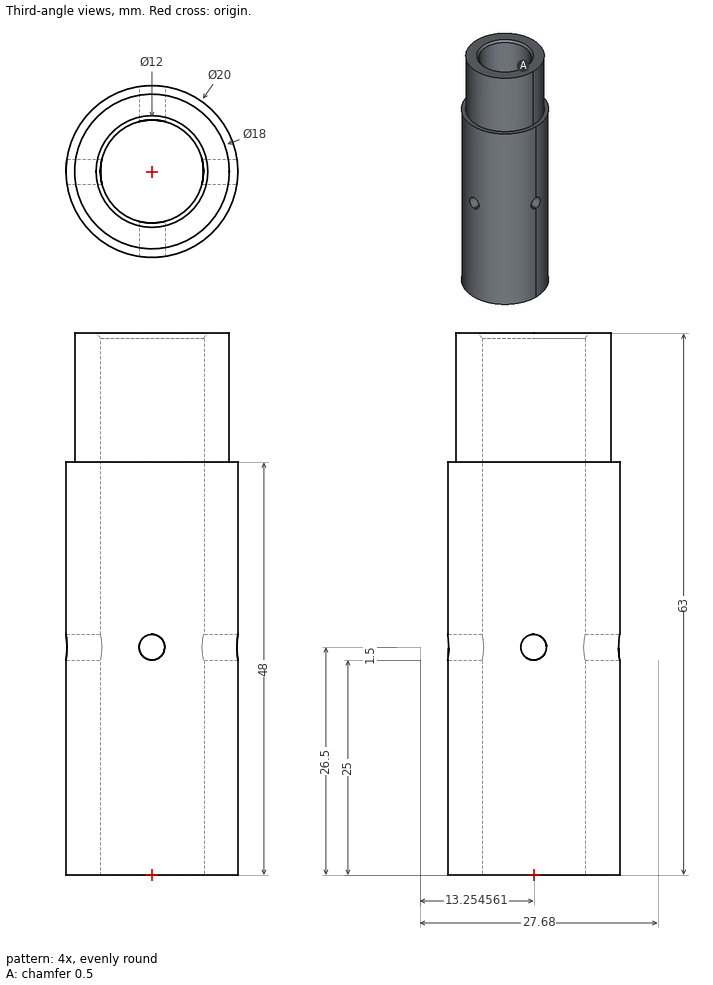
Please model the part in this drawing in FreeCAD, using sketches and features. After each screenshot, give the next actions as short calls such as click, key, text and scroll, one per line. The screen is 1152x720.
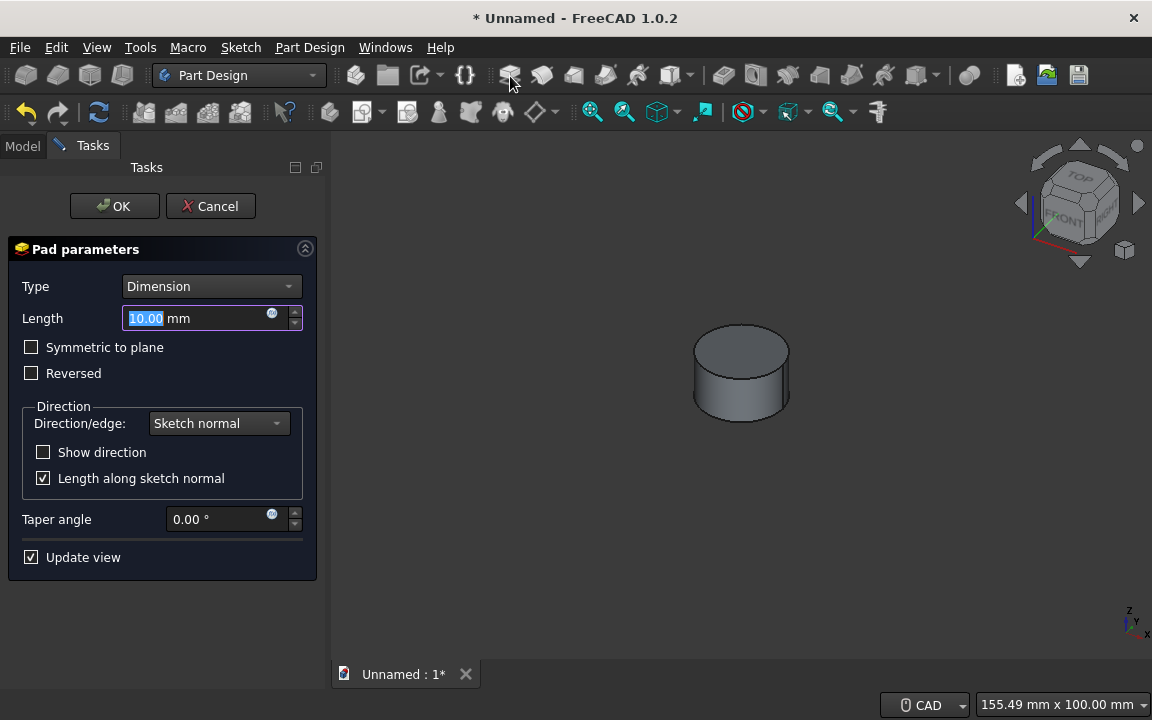
text(63)
key(Tab)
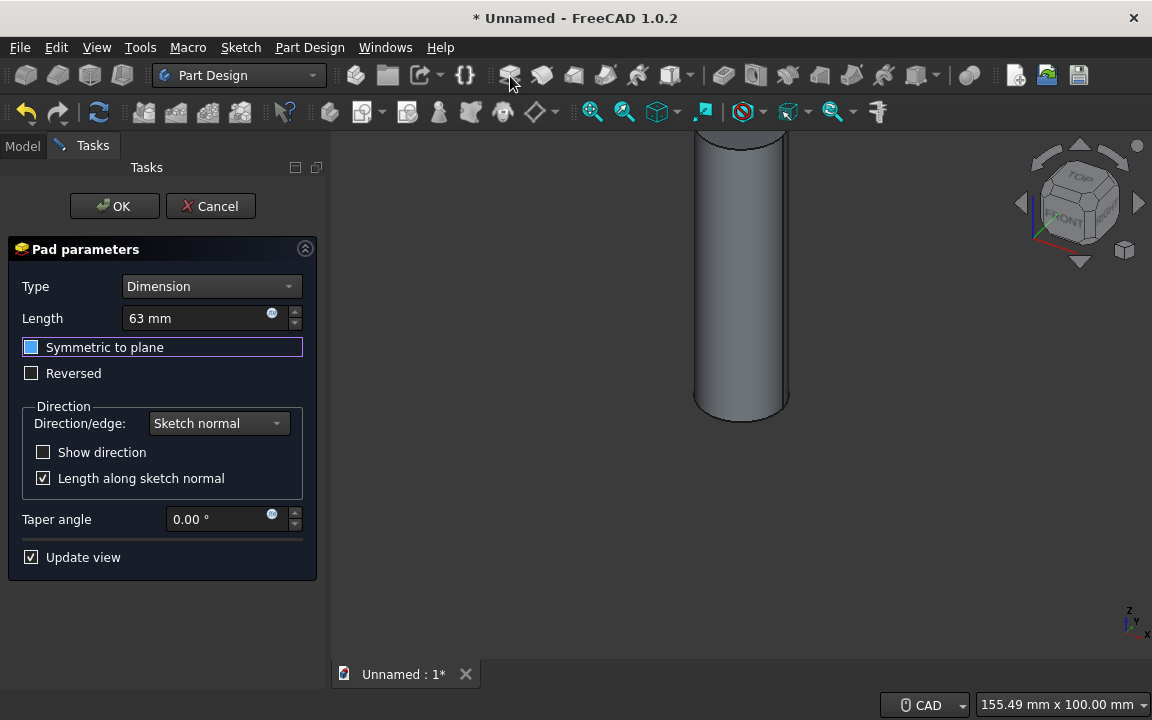
click(115, 206)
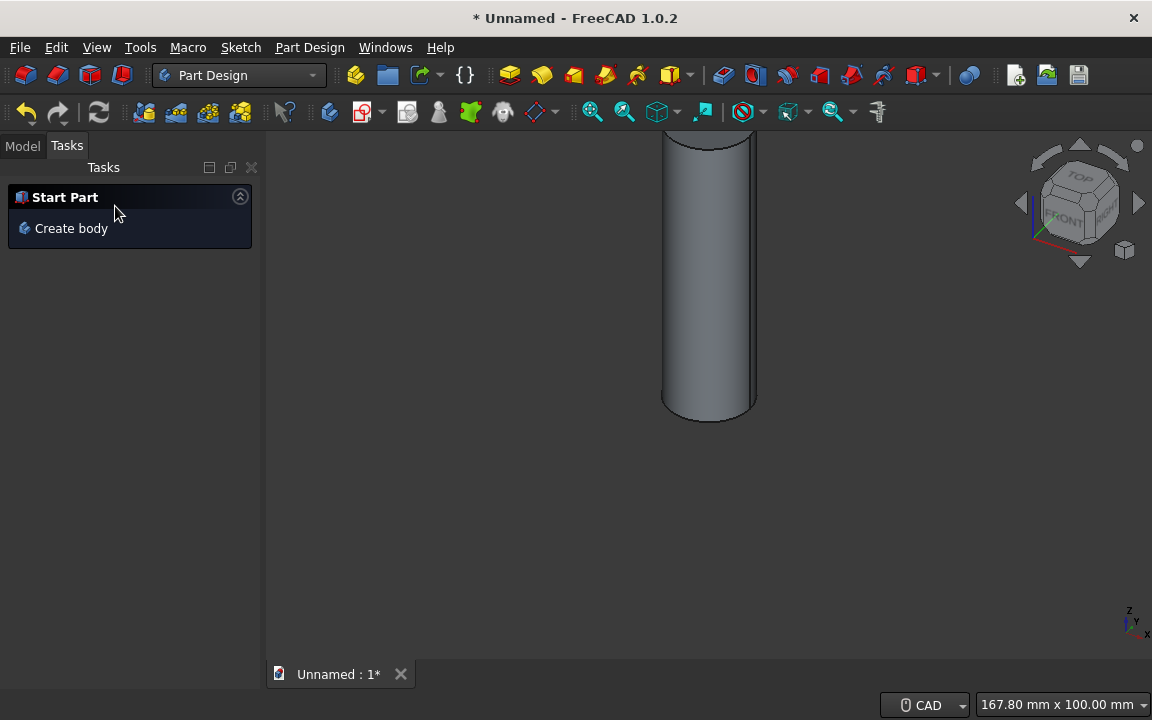
click(594, 112)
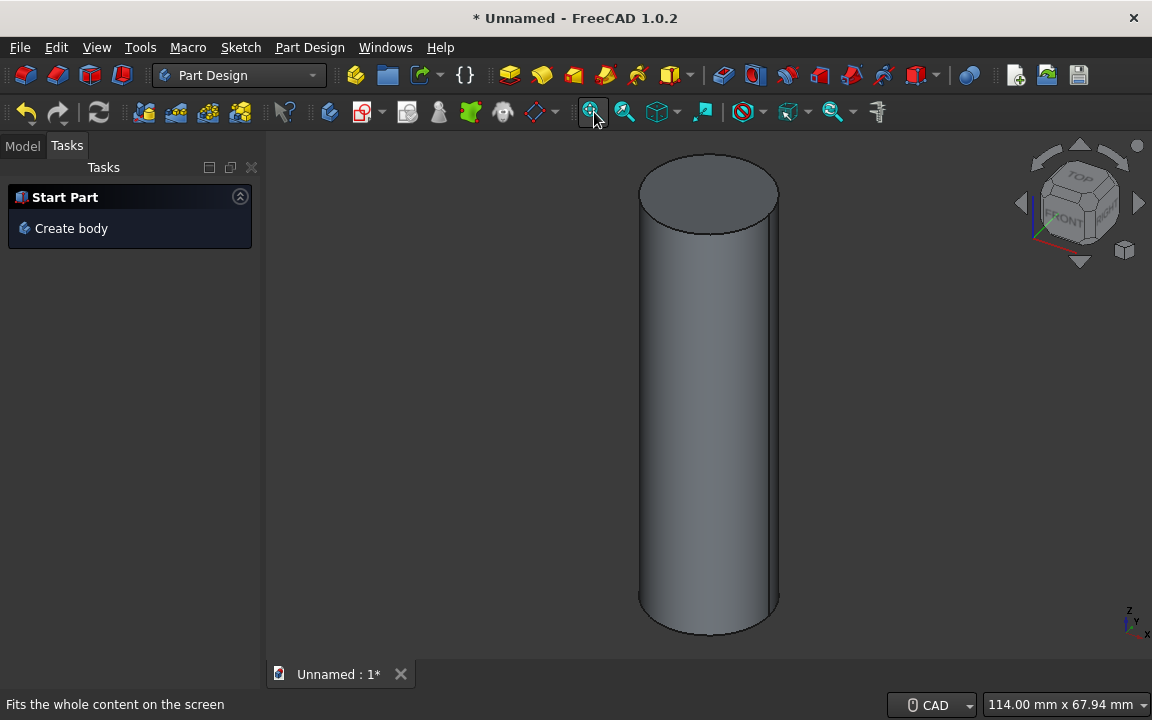
click(362, 112)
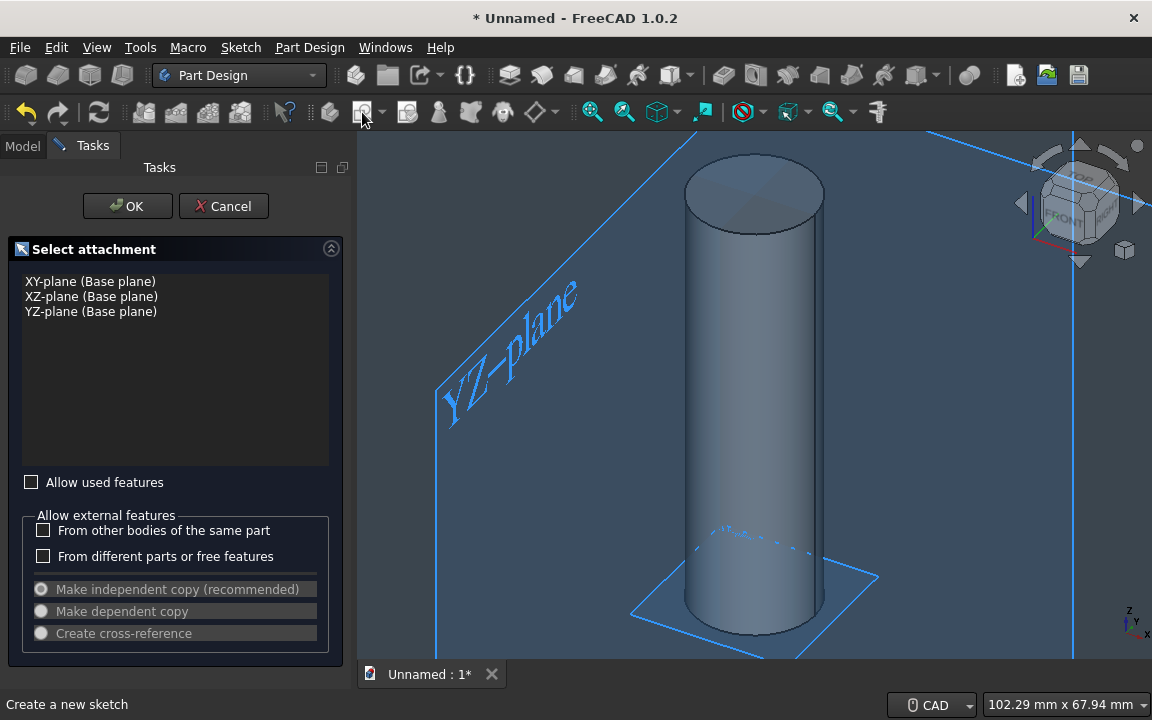
click(82, 282)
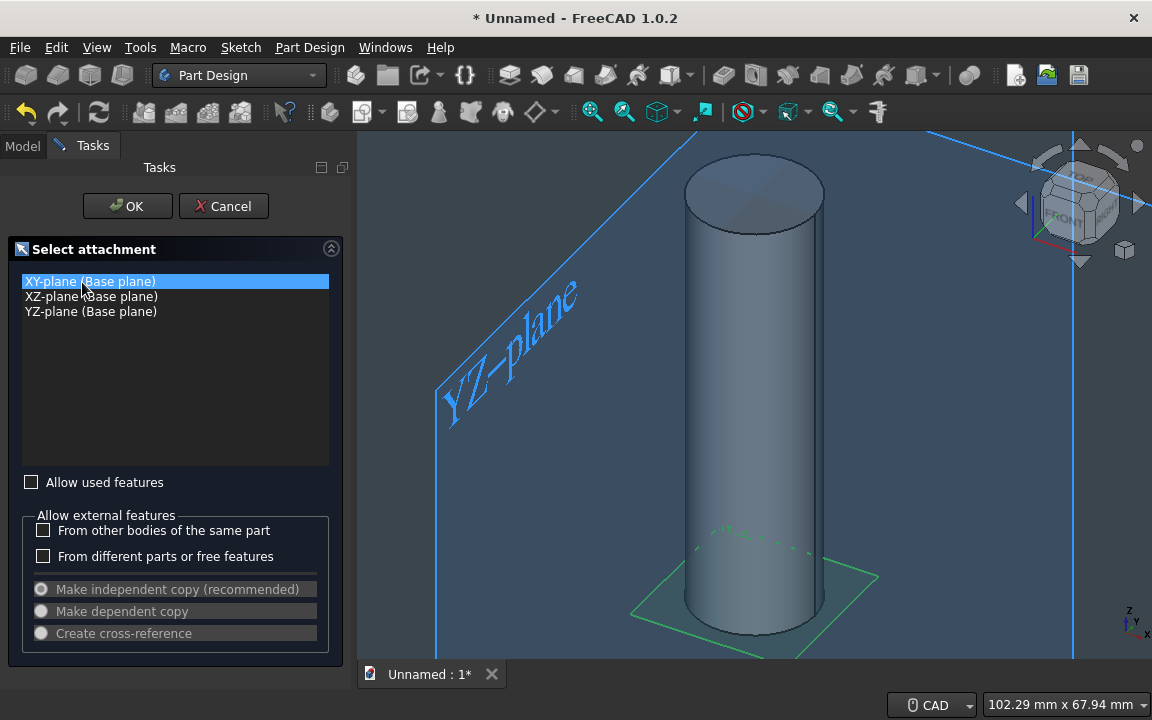
click(128, 206)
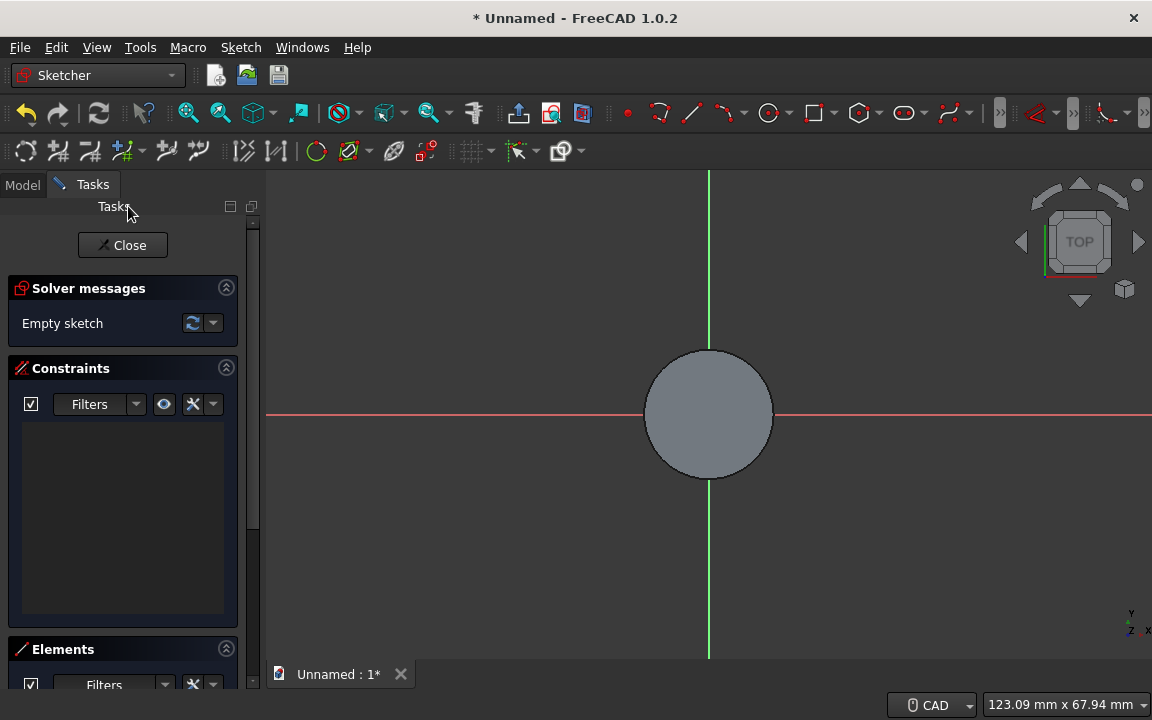
click(584, 114)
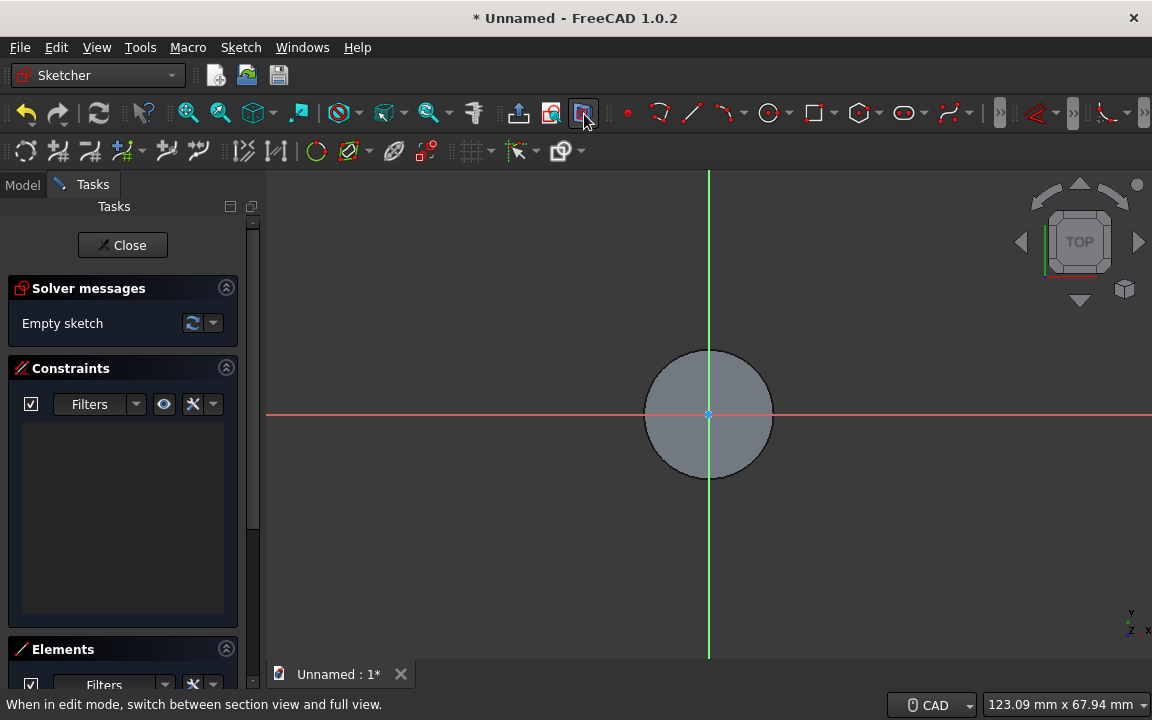
scroll(765, 414, up, 4)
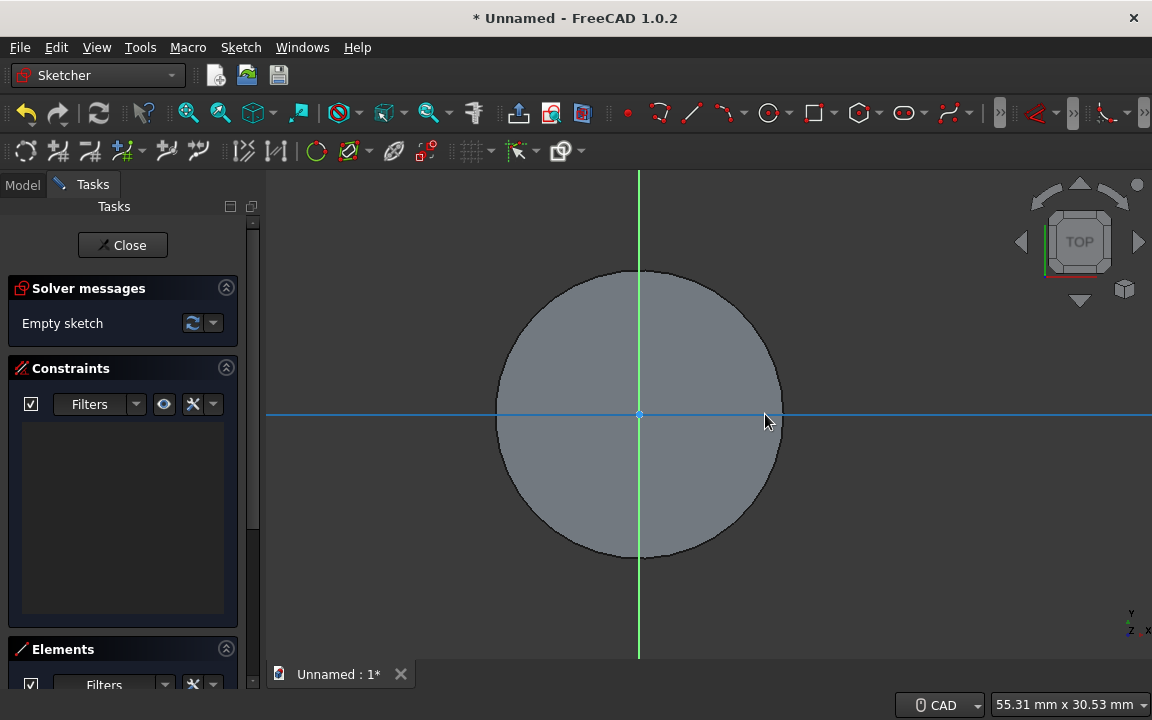
click(770, 114)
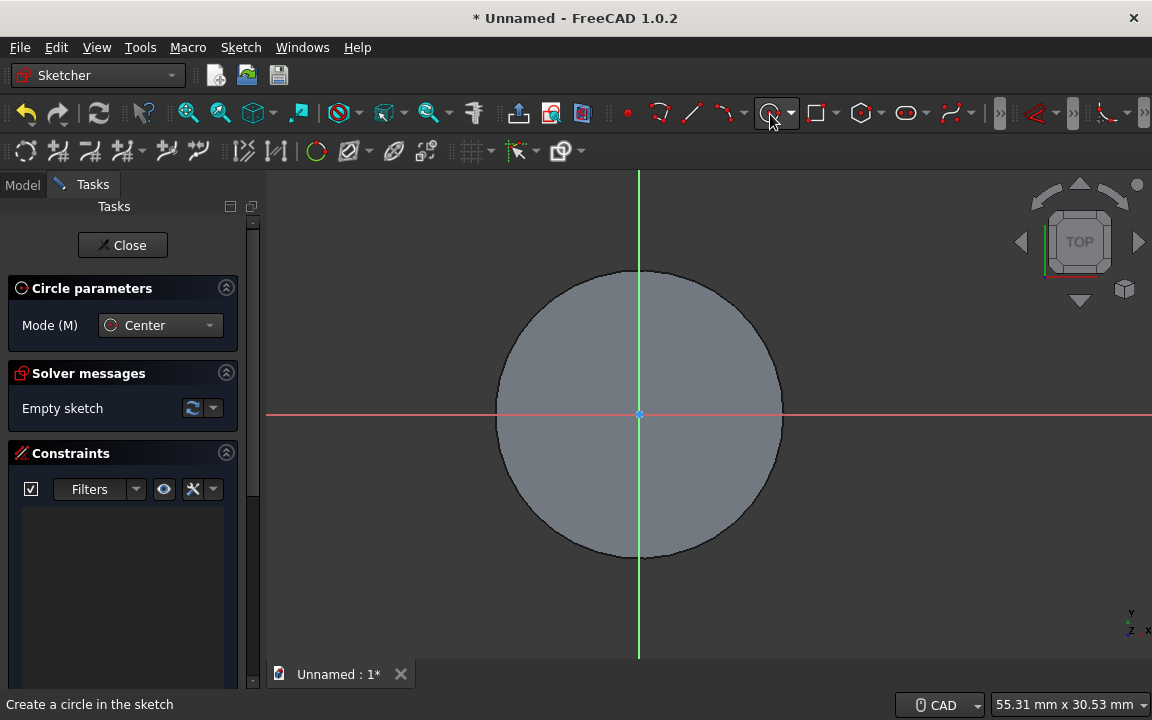
click(639, 414)
click(753, 301)
key(Escape)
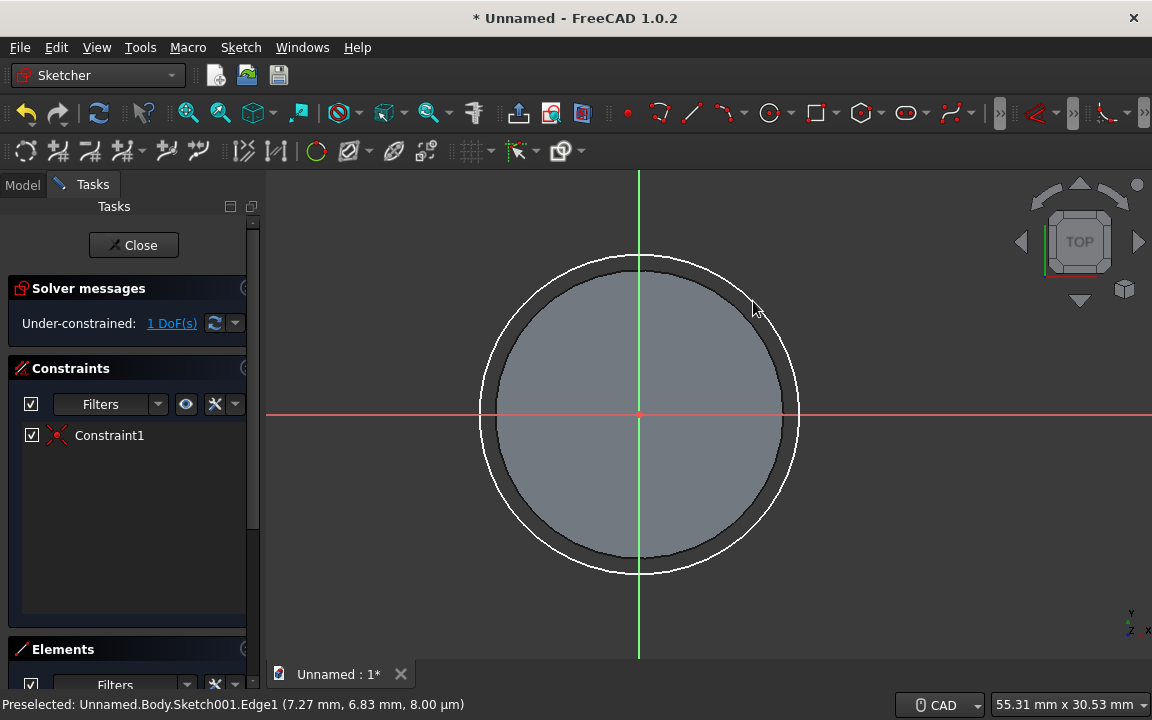
click(1036, 114)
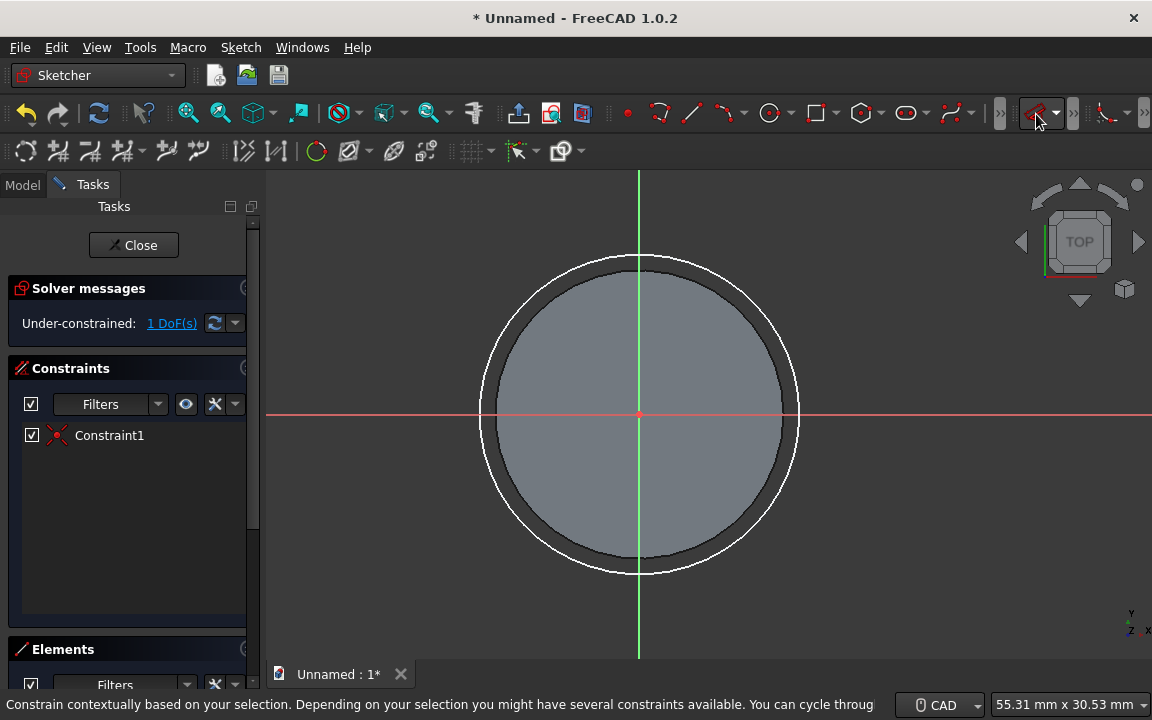
click(752, 301)
click(775, 278)